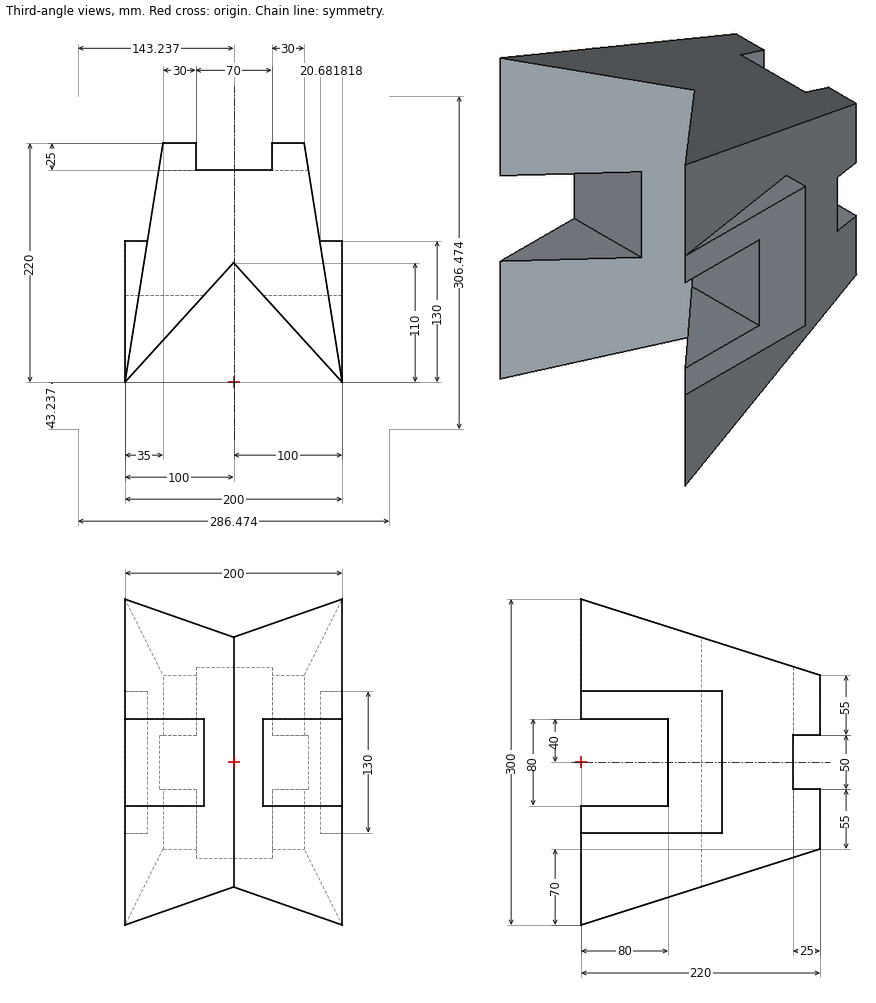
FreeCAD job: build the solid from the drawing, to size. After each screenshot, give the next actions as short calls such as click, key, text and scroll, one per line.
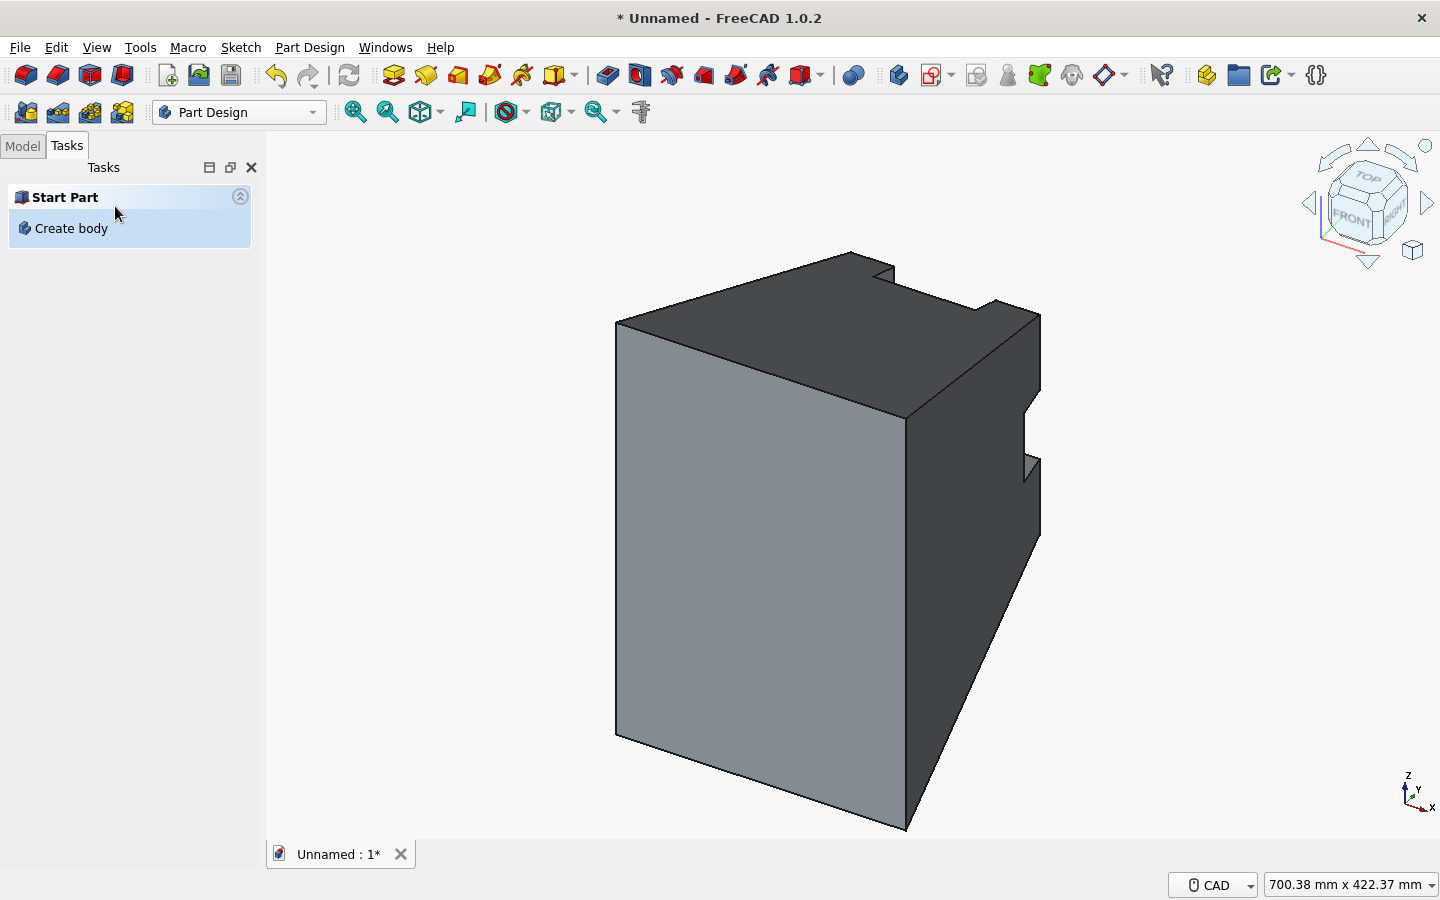
click(932, 76)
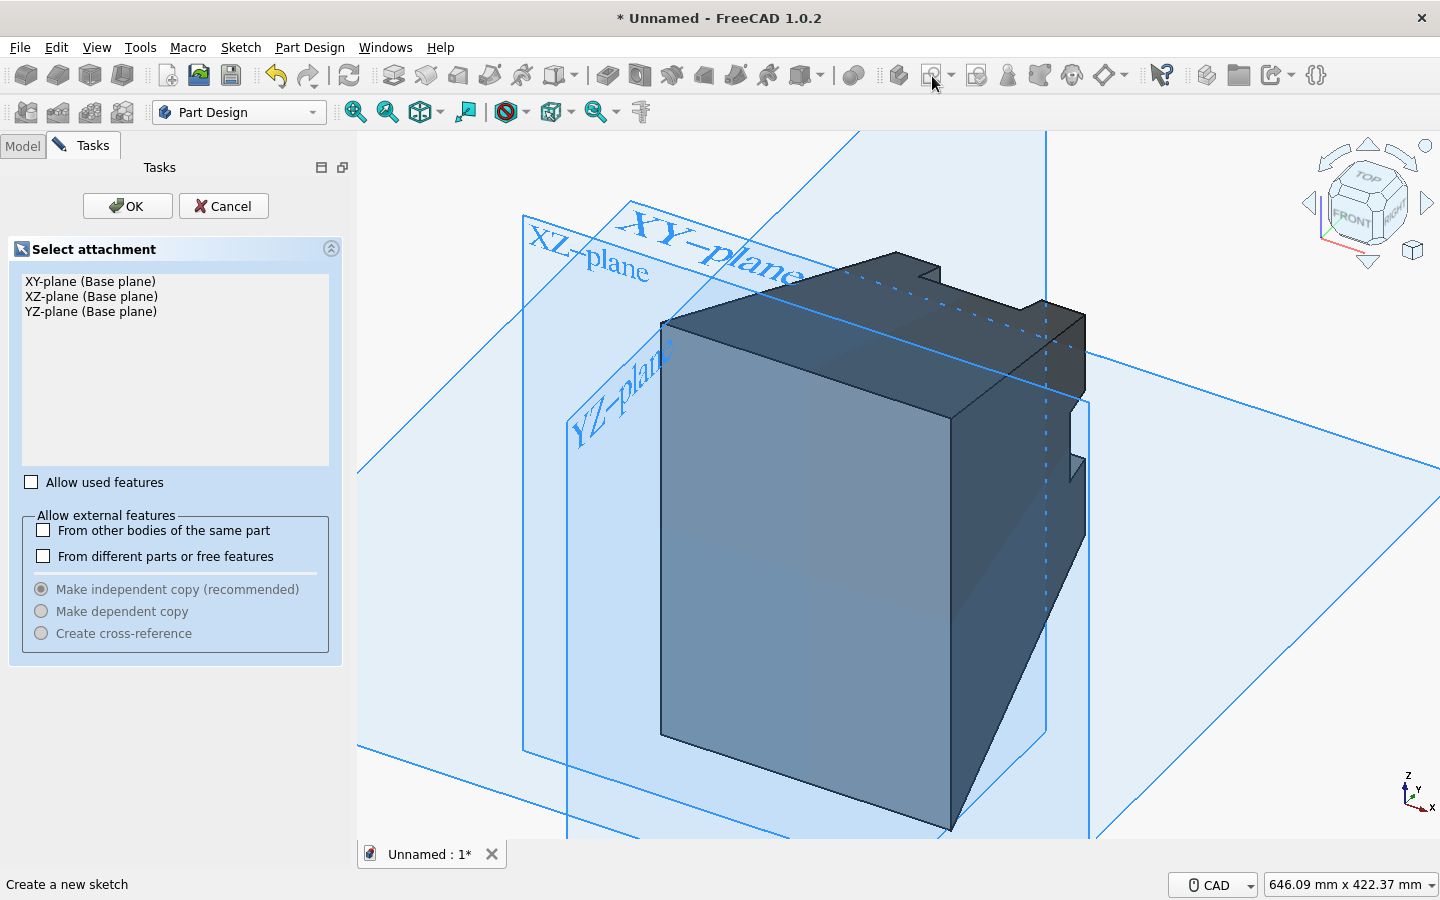
click(82, 282)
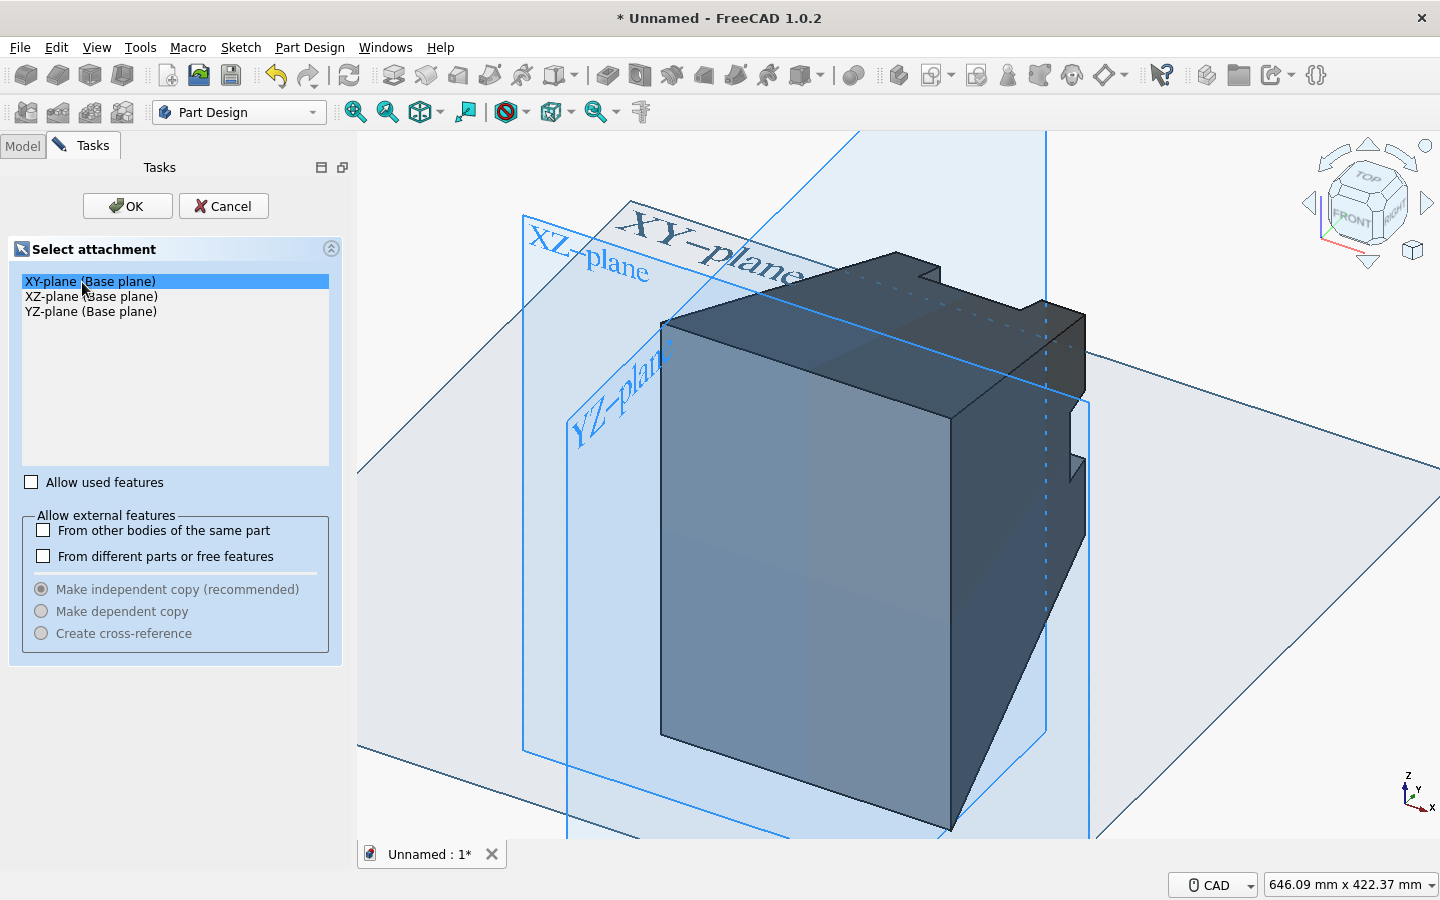
click(128, 206)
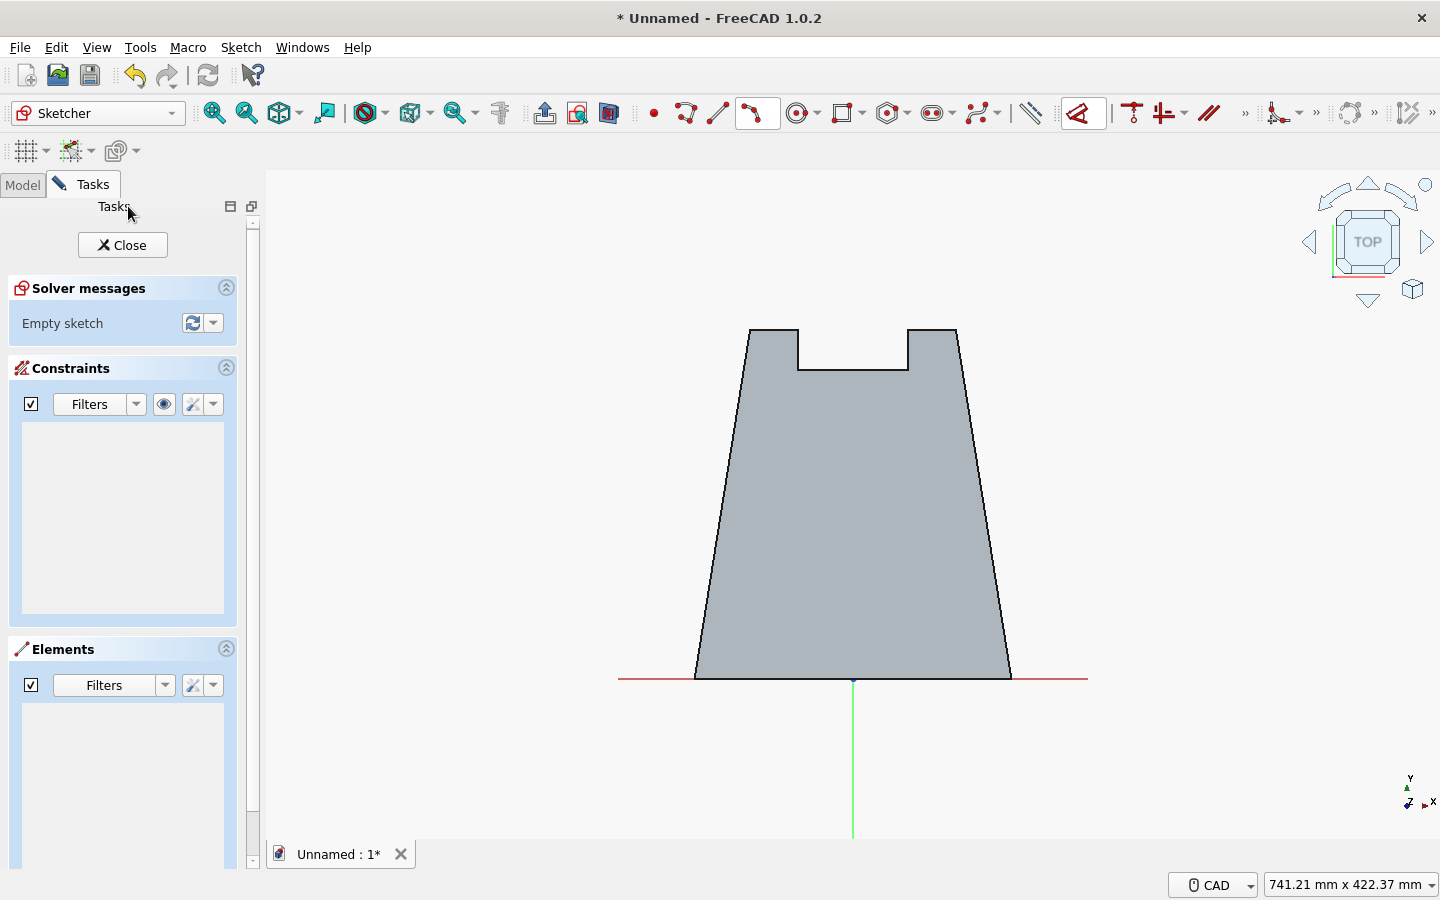
key(q)
key(s)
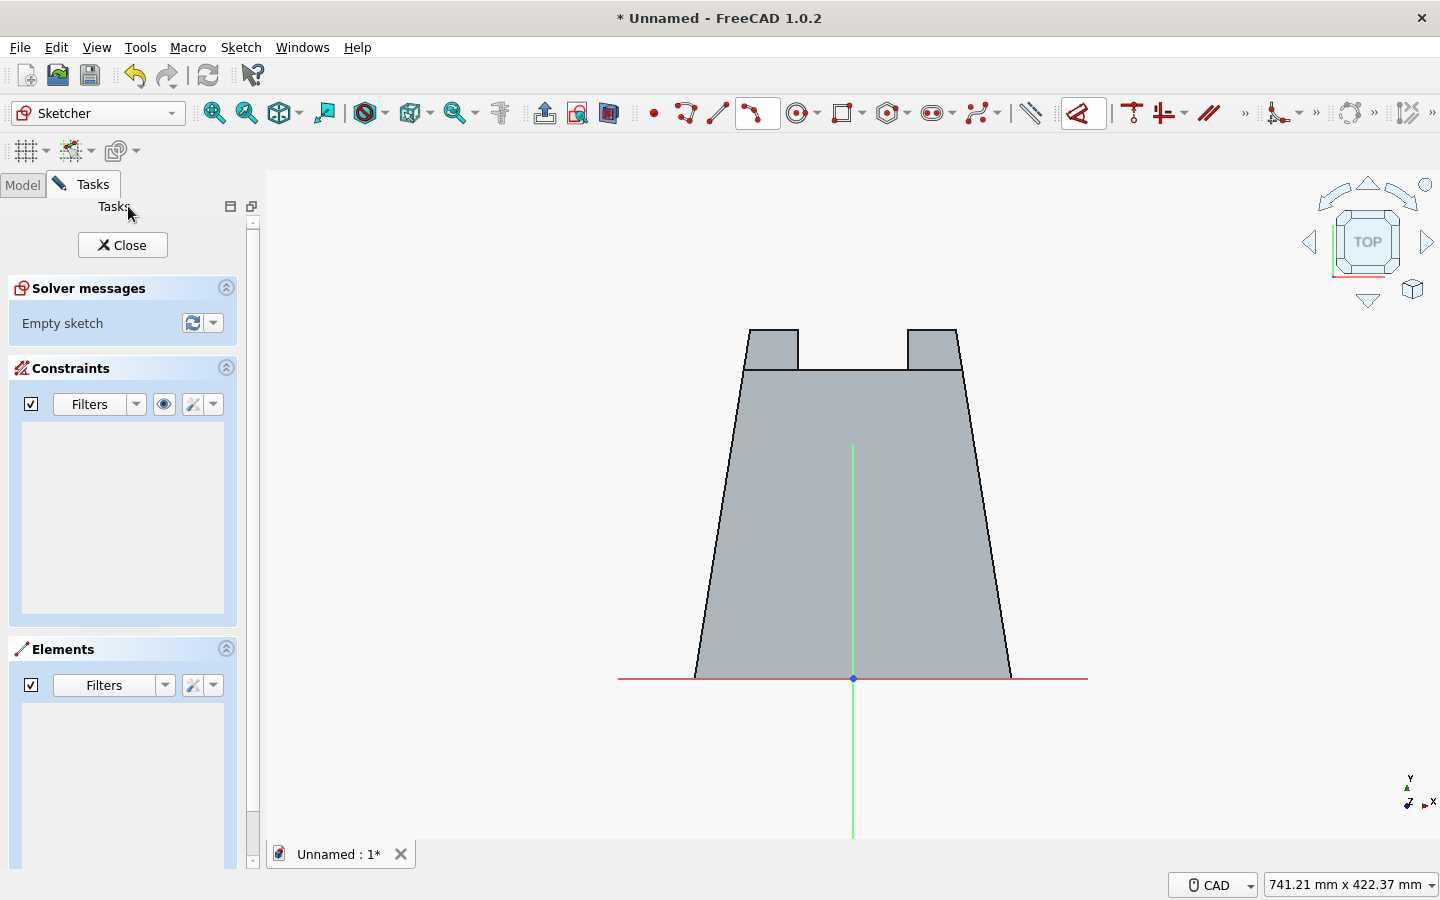
scroll(909, 663, up, 4)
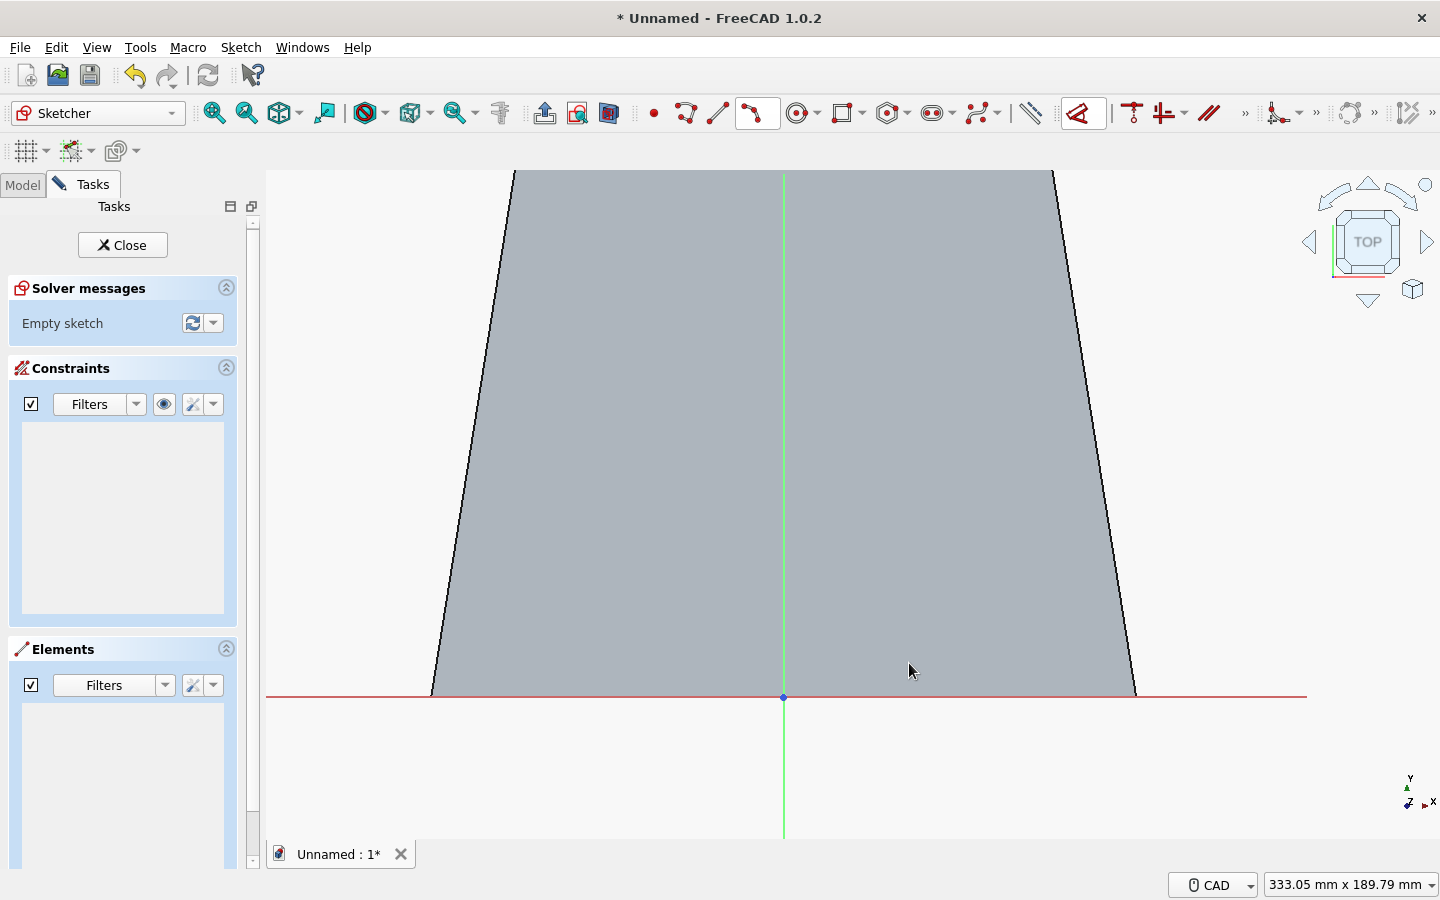
click(686, 114)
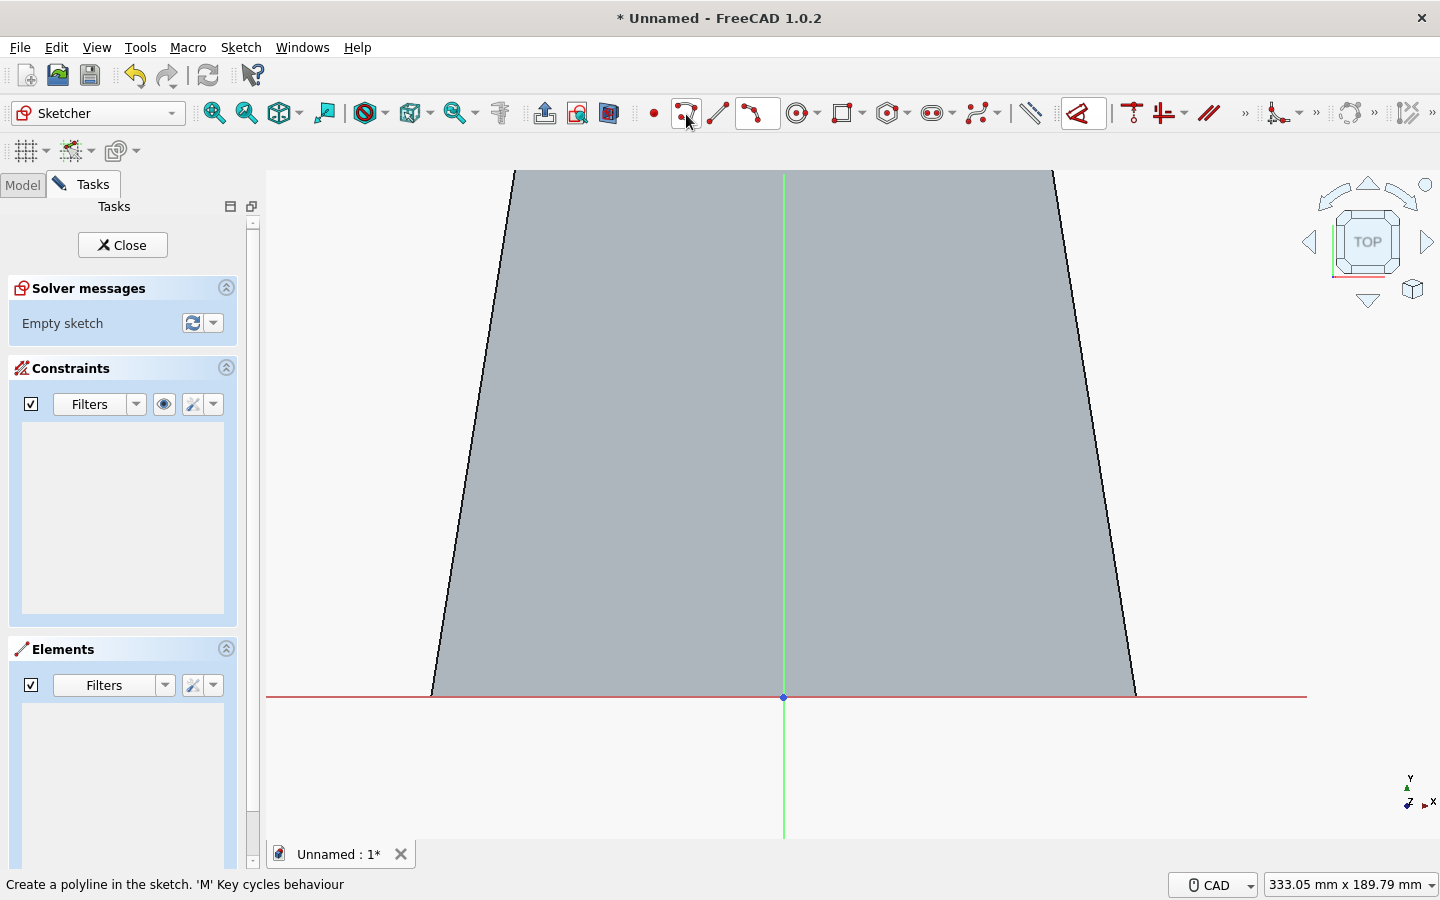
click(431, 697)
click(1136, 688)
click(784, 309)
click(431, 697)
key(Escape)
key(Escape)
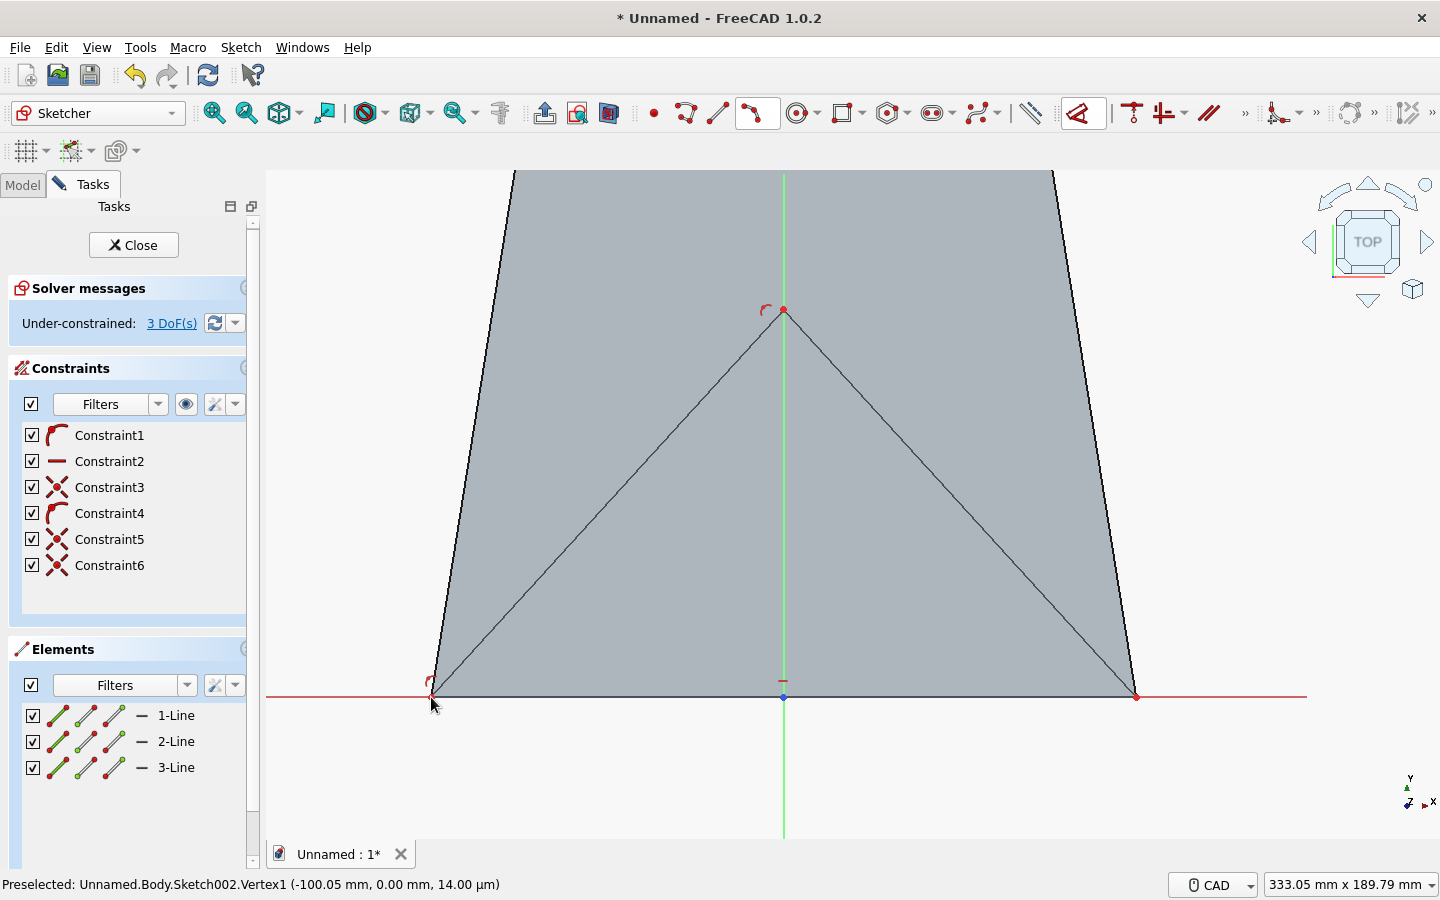
click(642, 697)